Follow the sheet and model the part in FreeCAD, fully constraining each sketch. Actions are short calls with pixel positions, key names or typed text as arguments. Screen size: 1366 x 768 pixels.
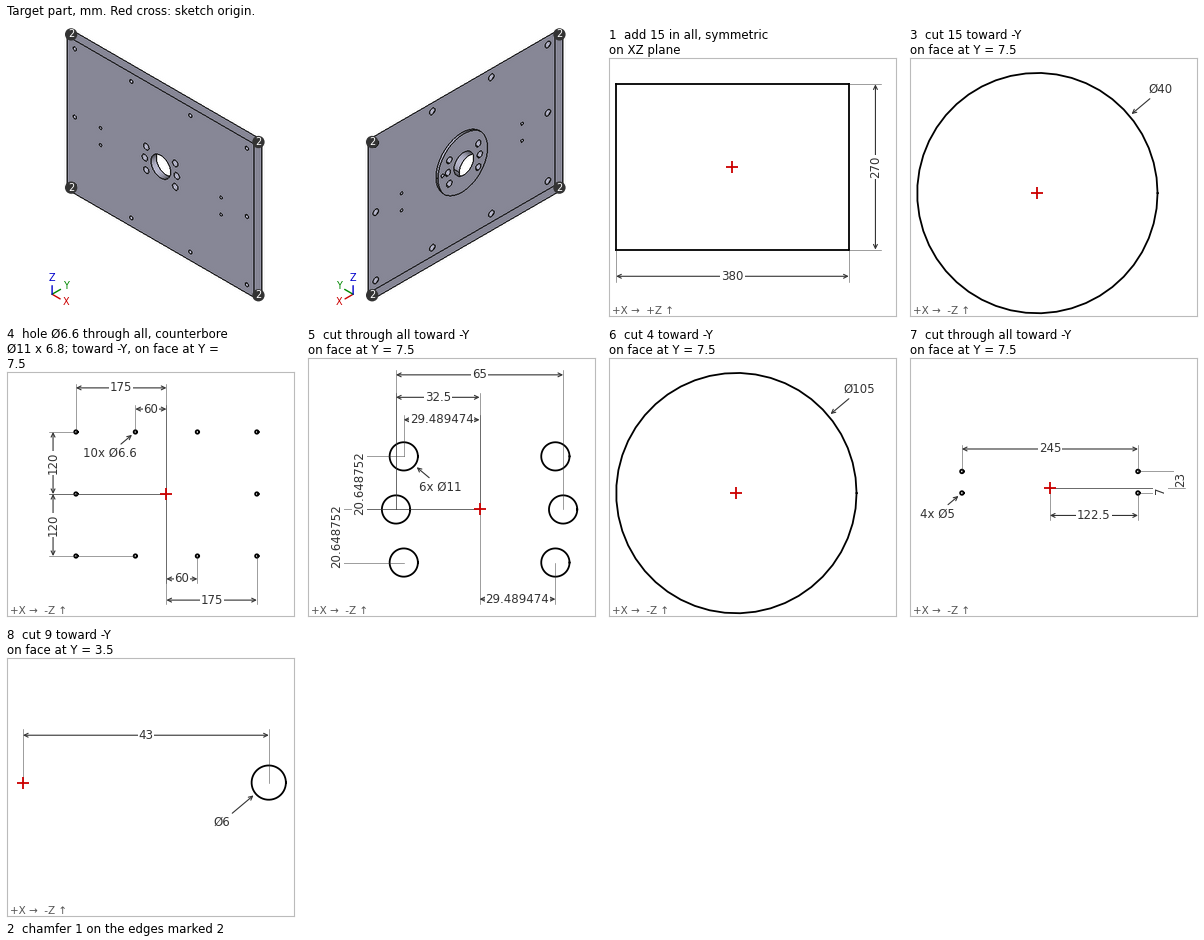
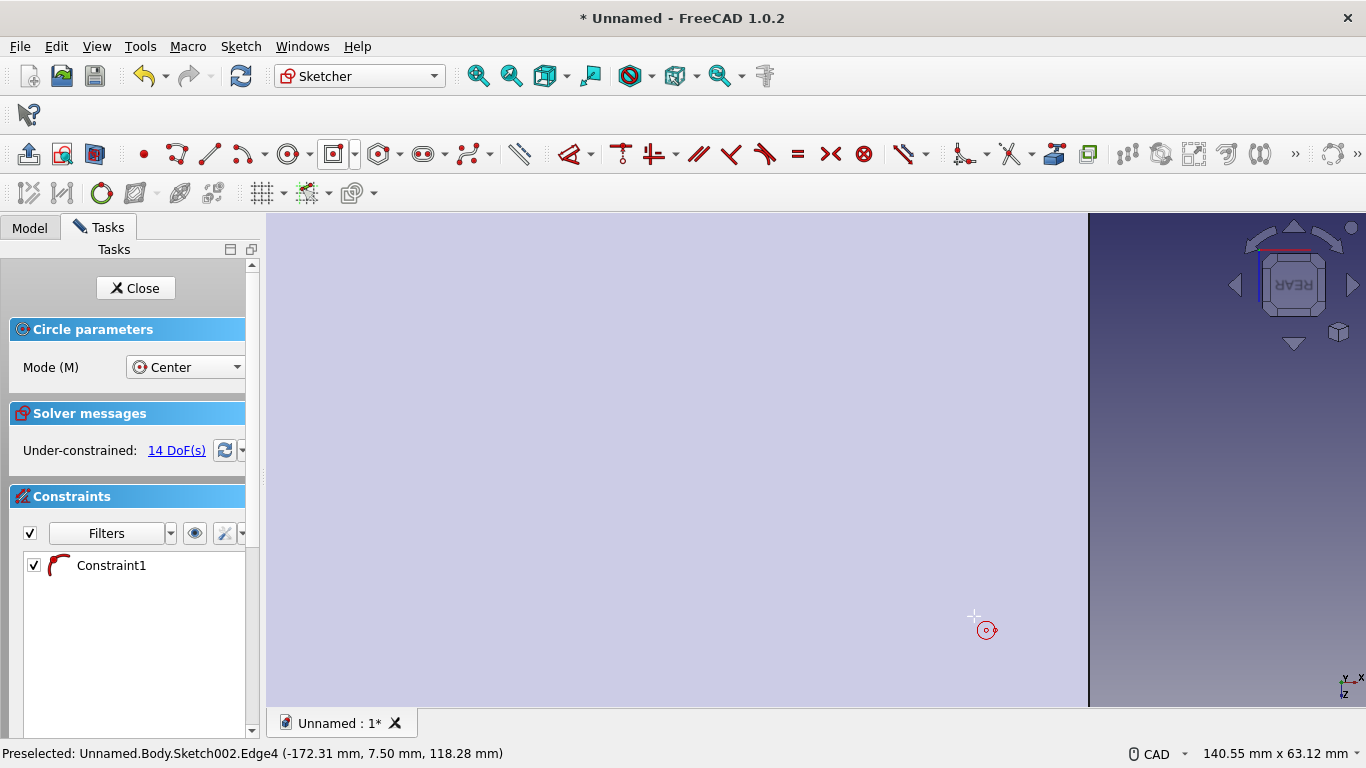
scroll(974, 616, down, 9)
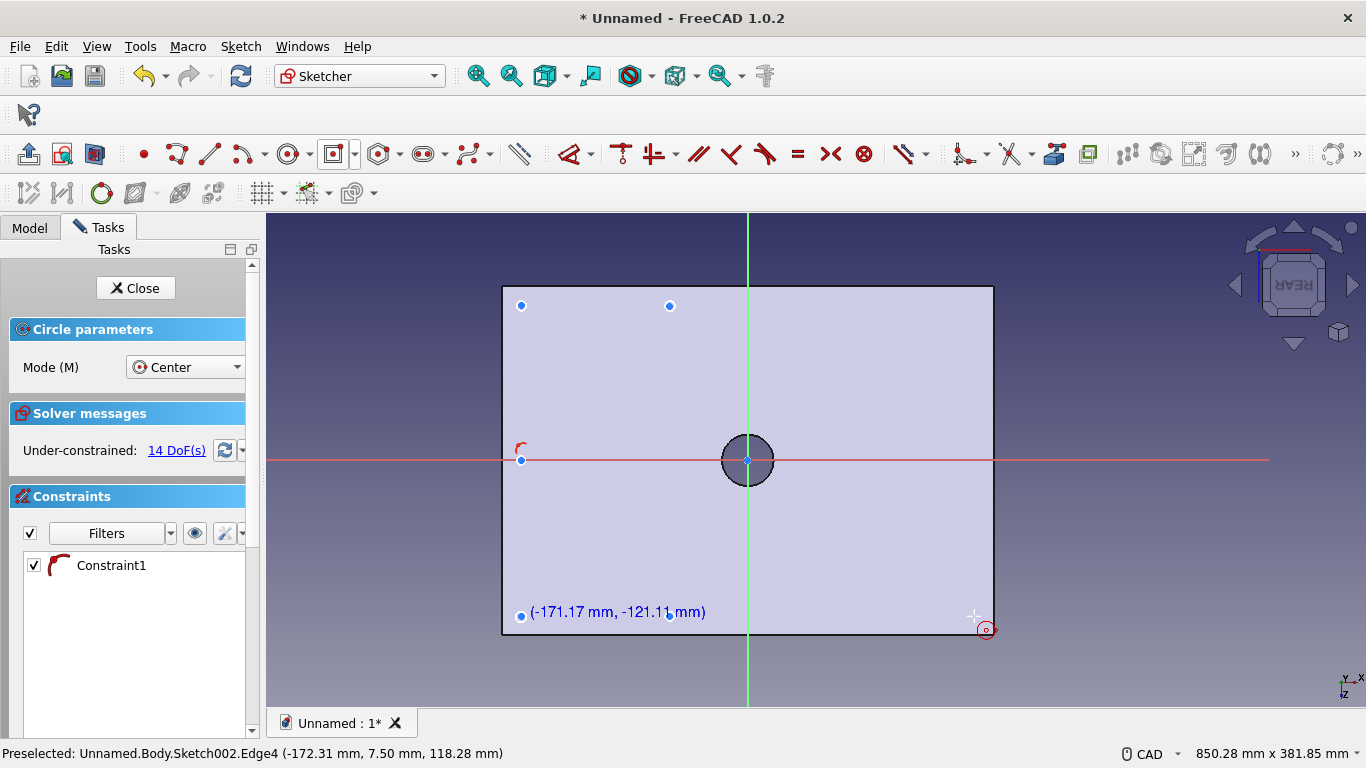
click(974, 616)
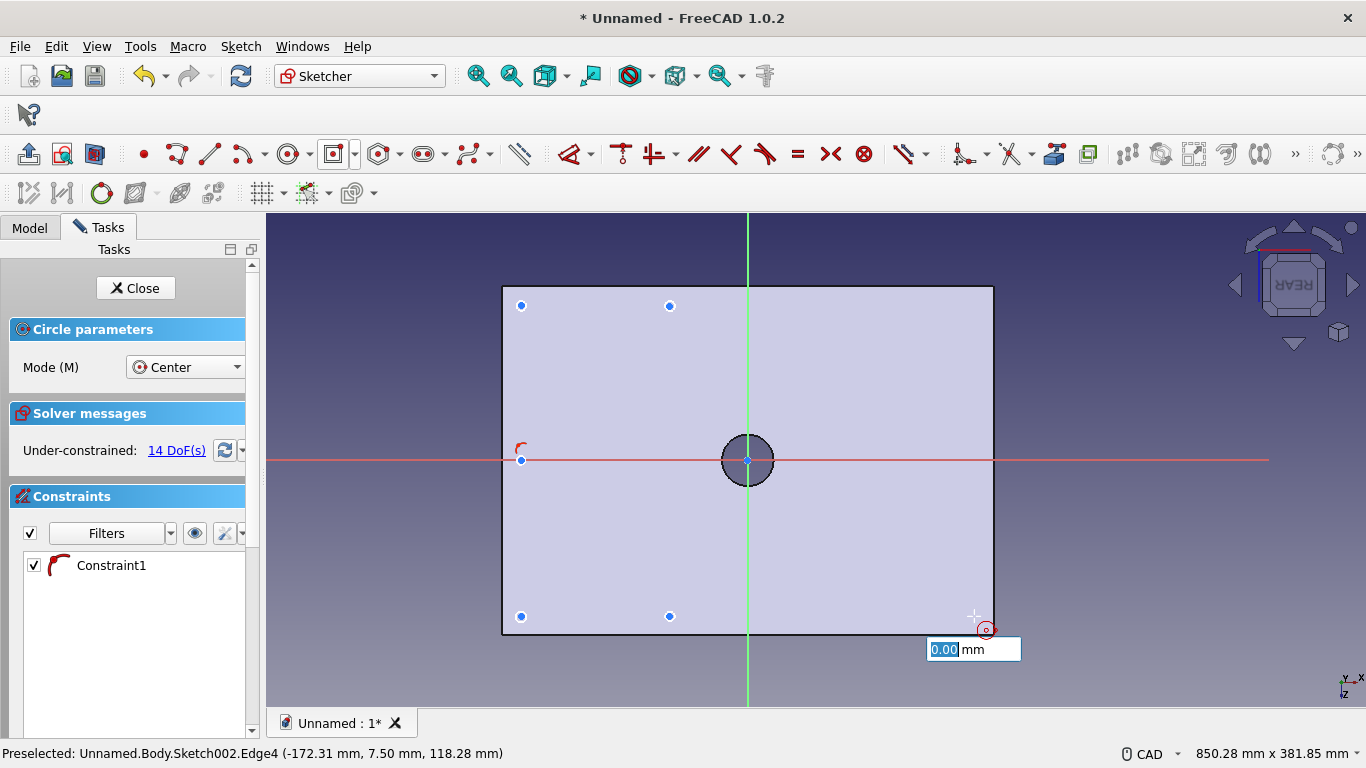
scroll(977, 613, up, 7)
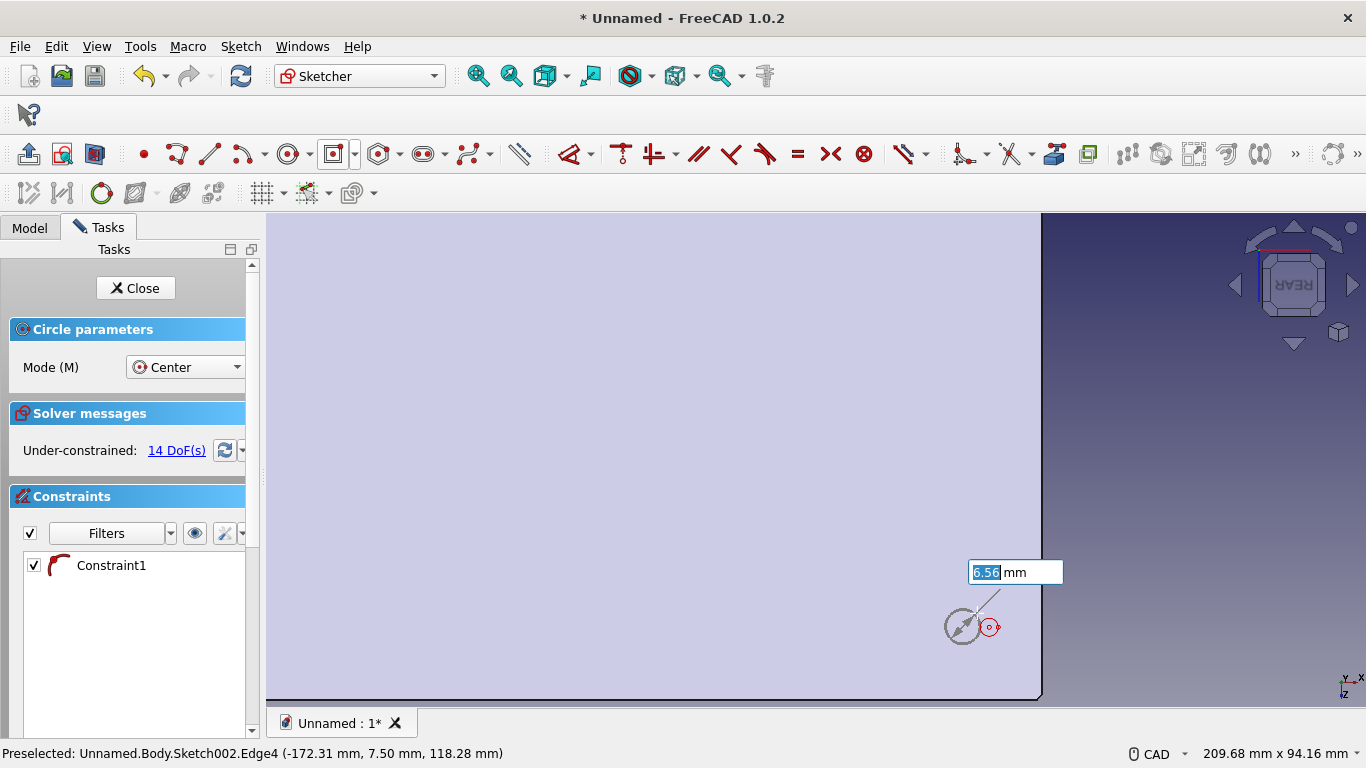
click(976, 609)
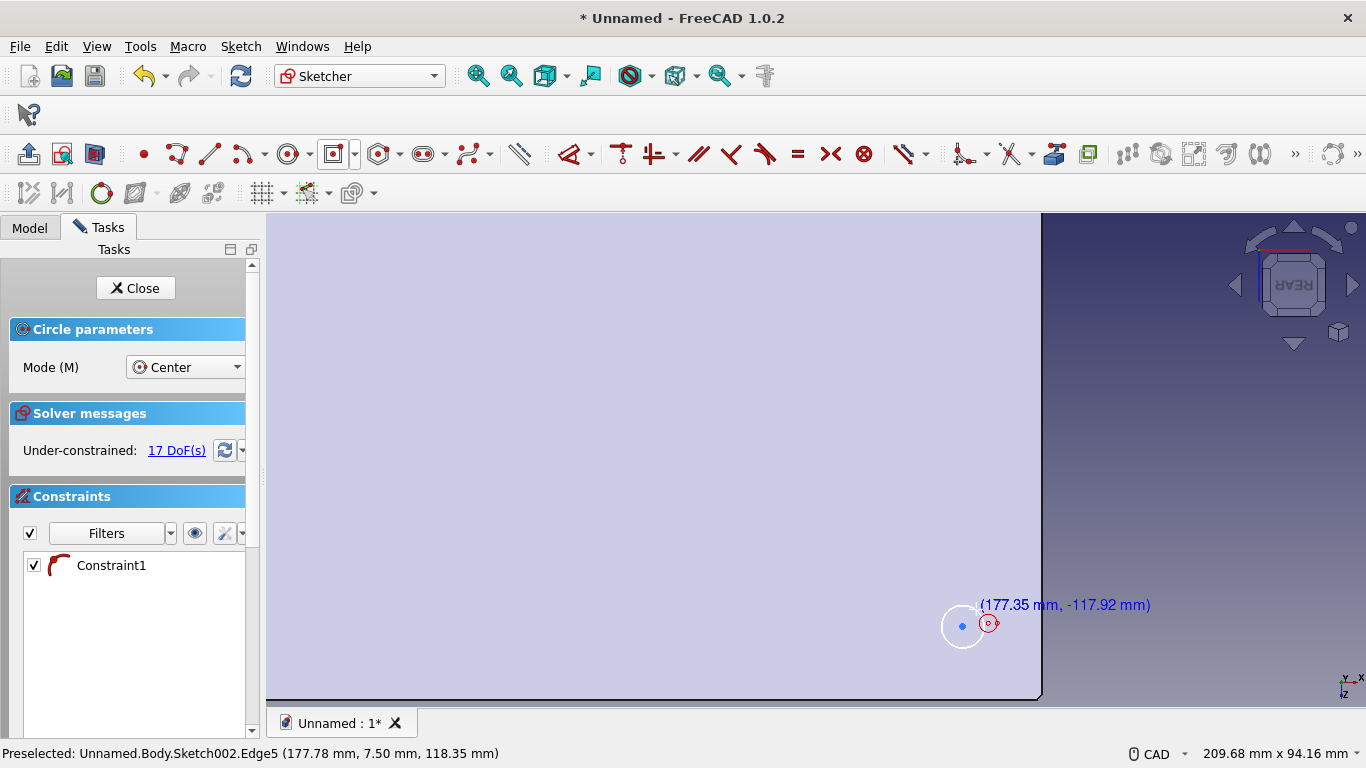
scroll(977, 613, down, 7)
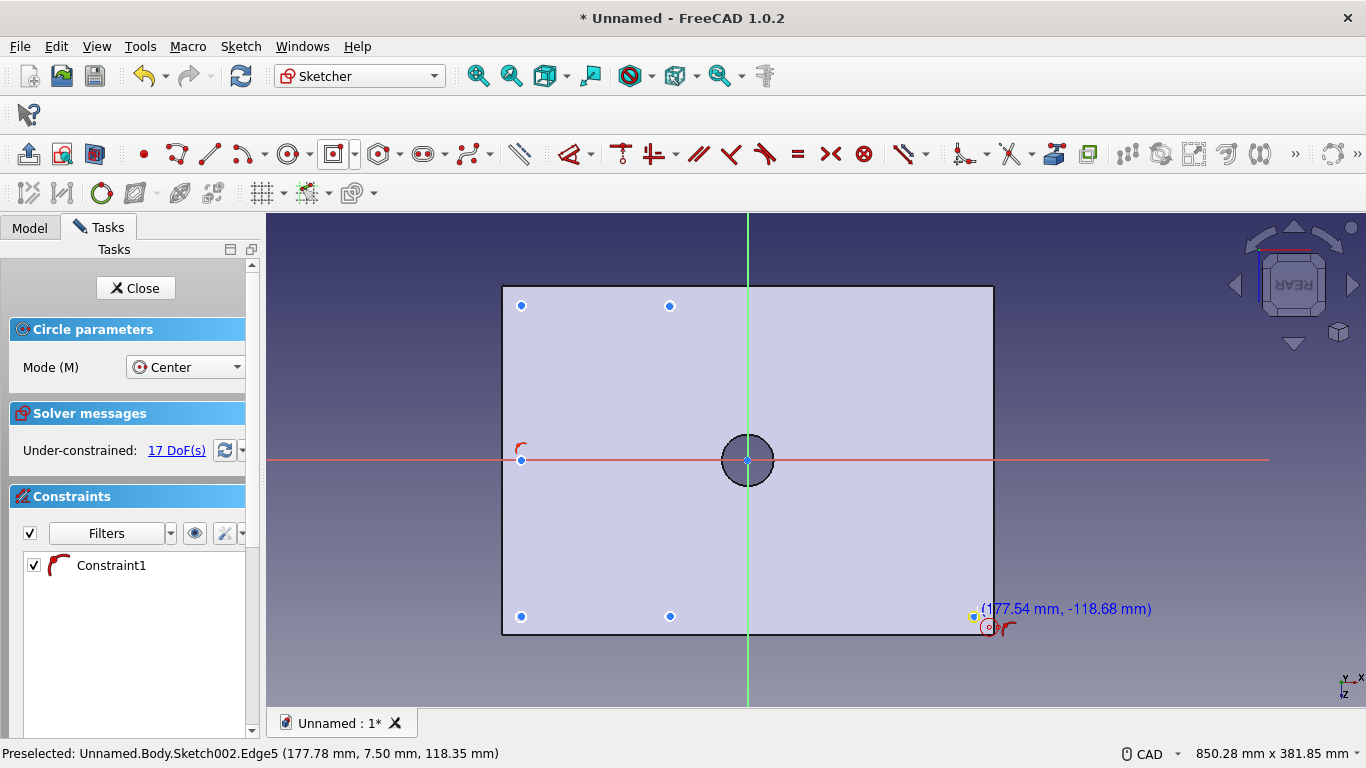
scroll(974, 460, up, 9)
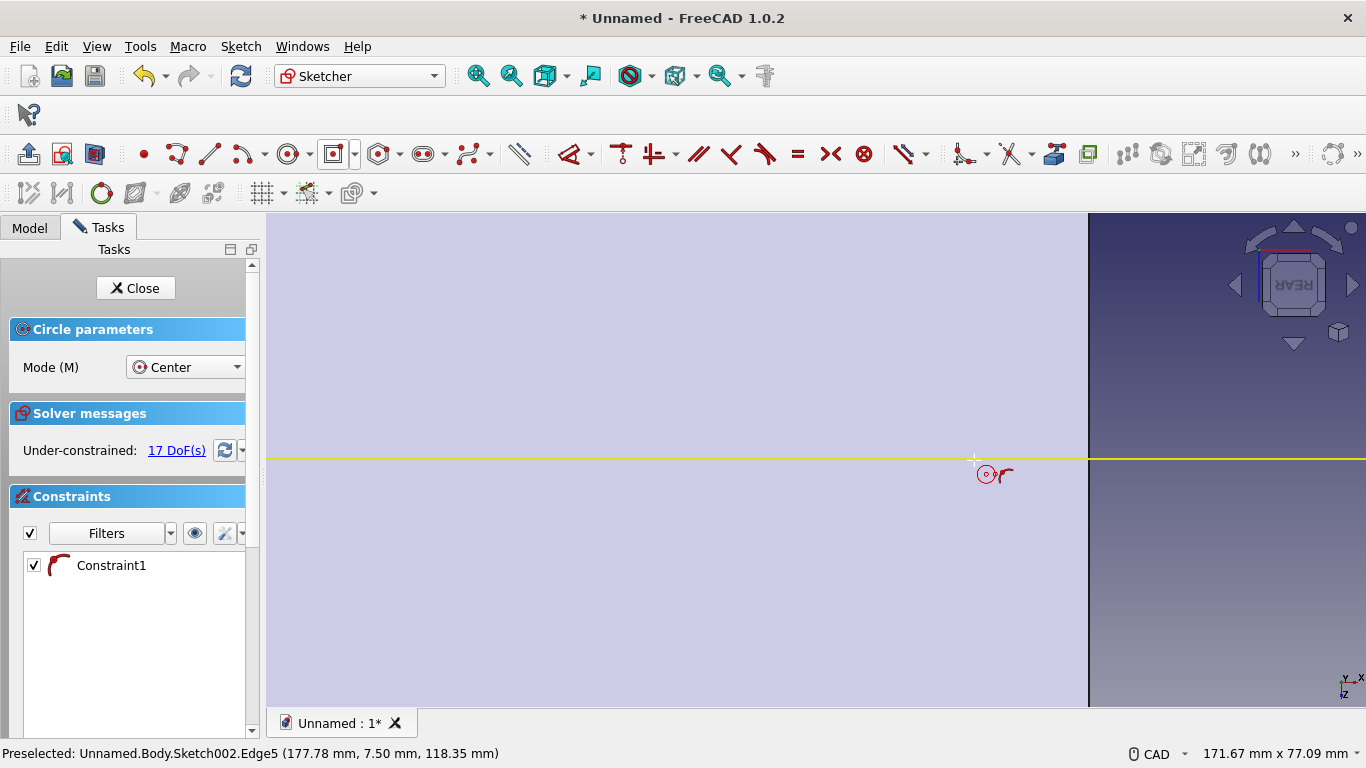
scroll(974, 460, down, 9)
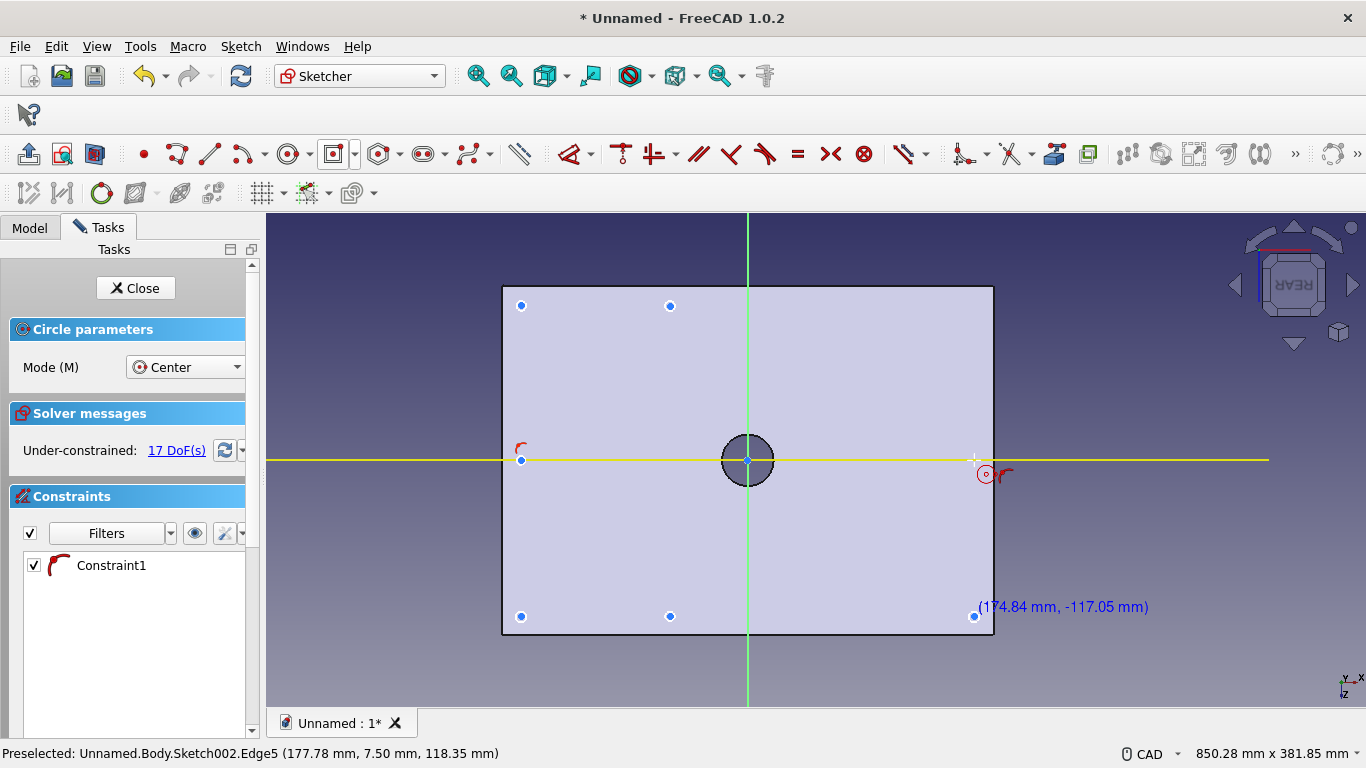
click(974, 460)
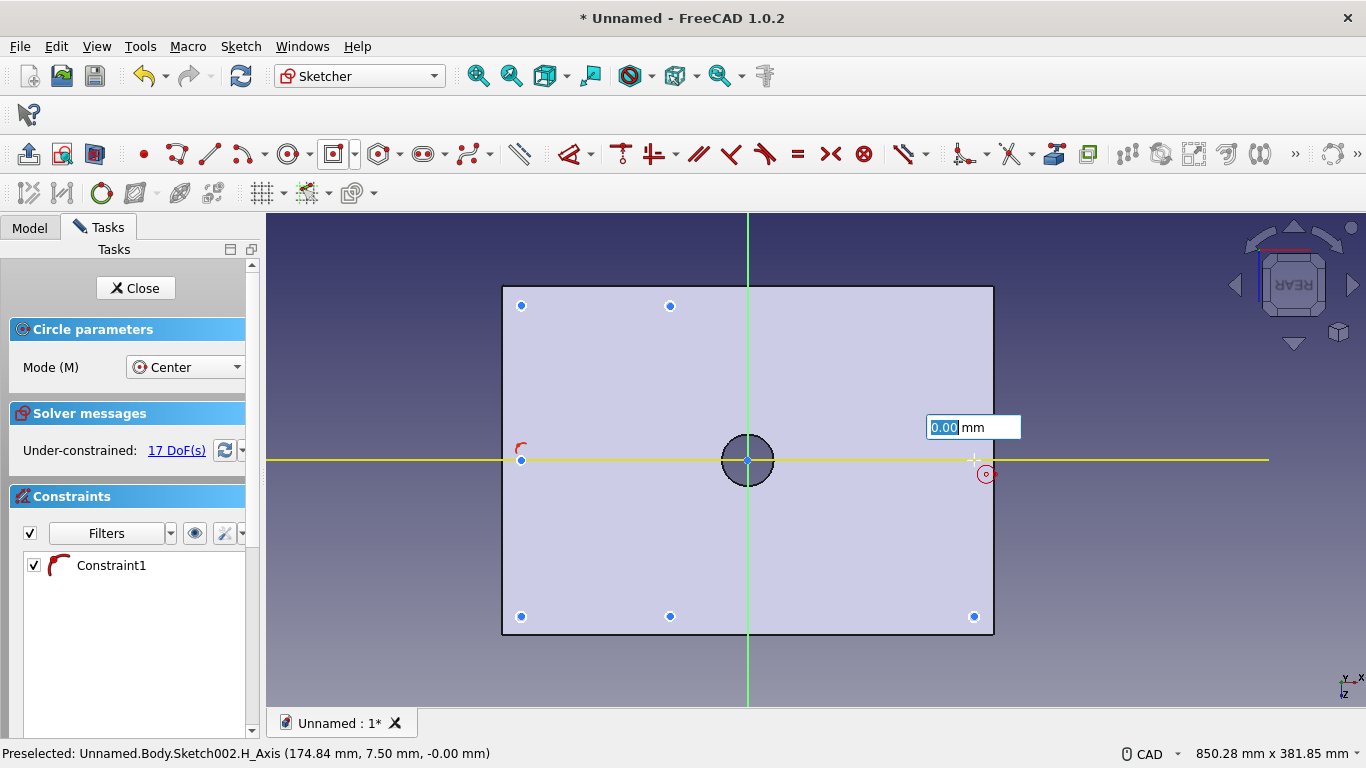
scroll(973, 464, up, 7)